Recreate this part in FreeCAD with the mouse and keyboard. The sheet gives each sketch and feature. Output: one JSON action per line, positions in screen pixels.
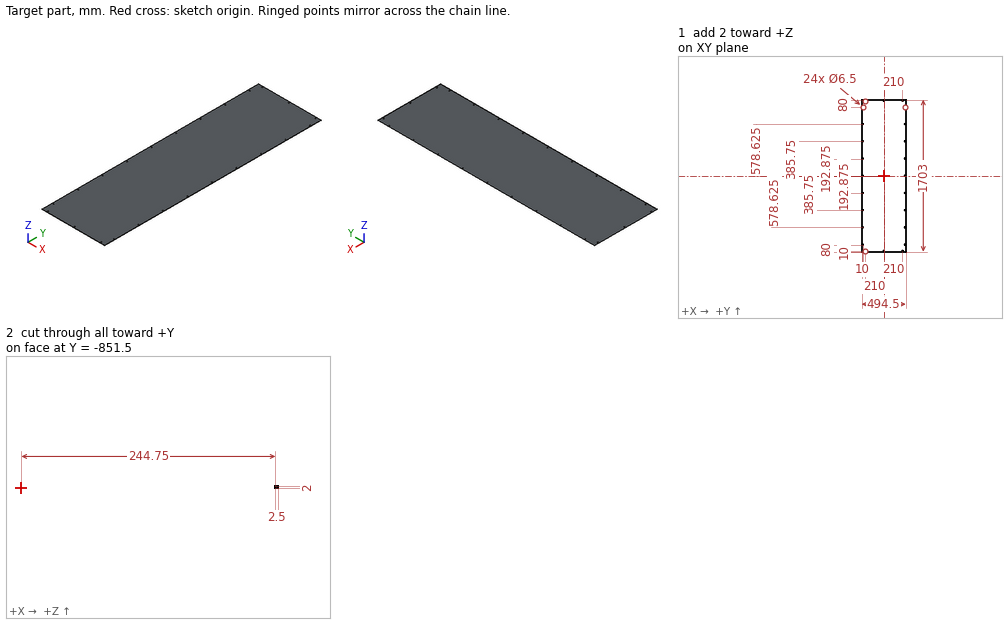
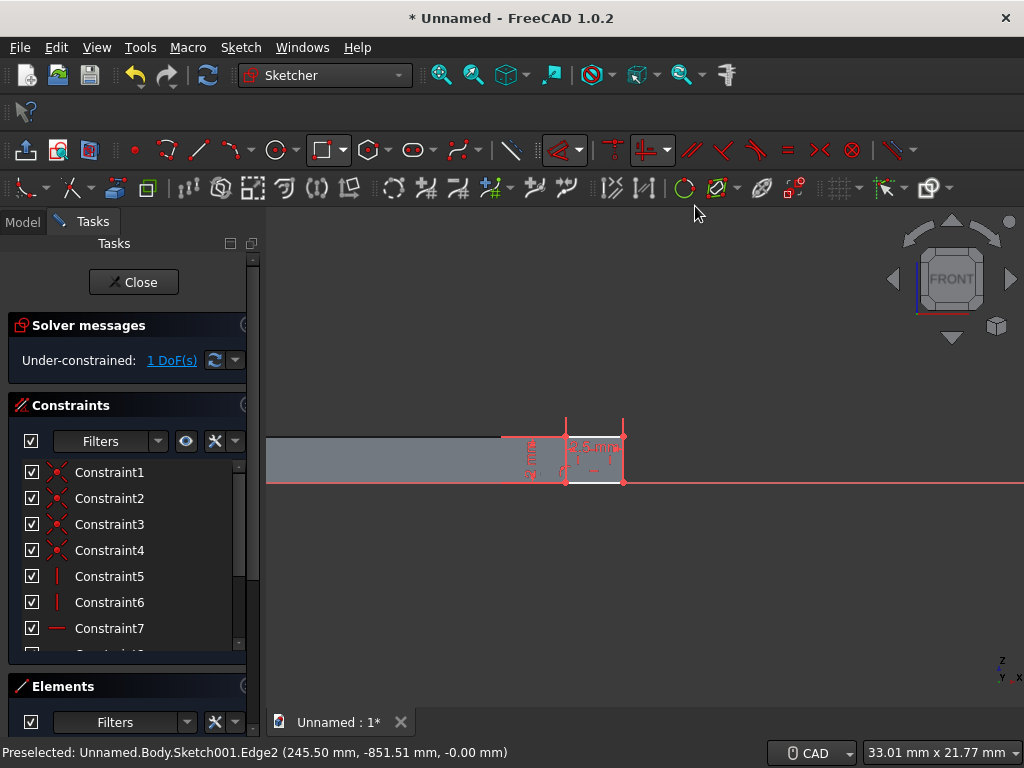
{"action": "scroll", "coordinate": [597, 460], "scroll_direction": "up", "scroll_amount": 10}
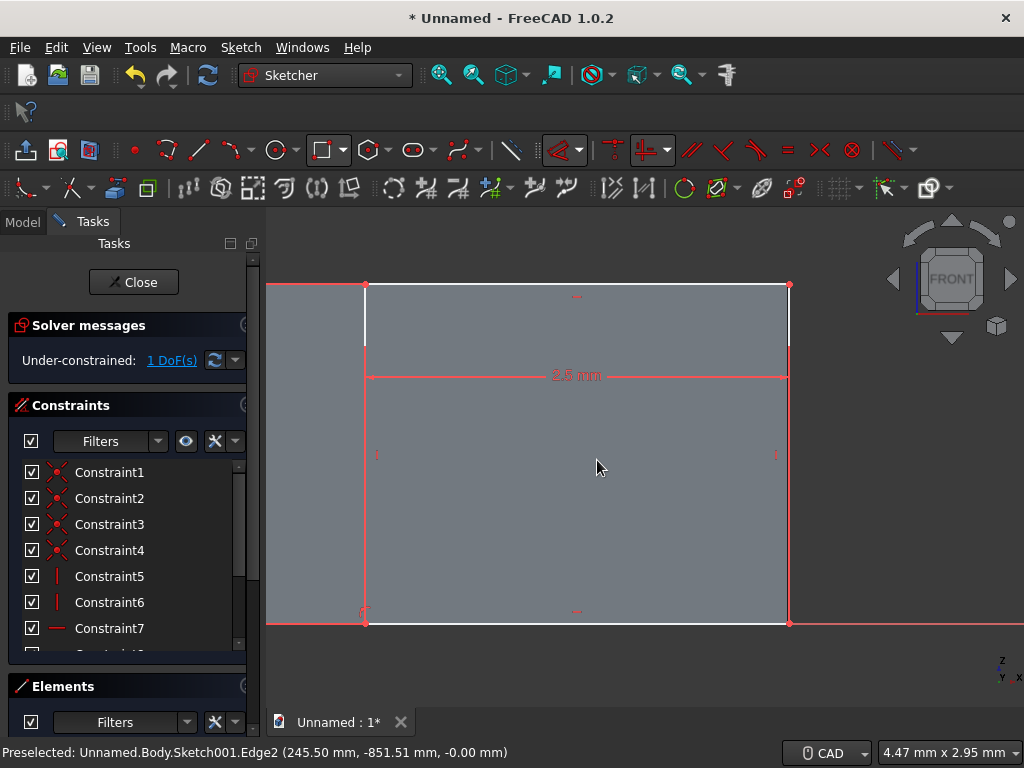
{"action": "left_click", "coordinate": [365, 284]}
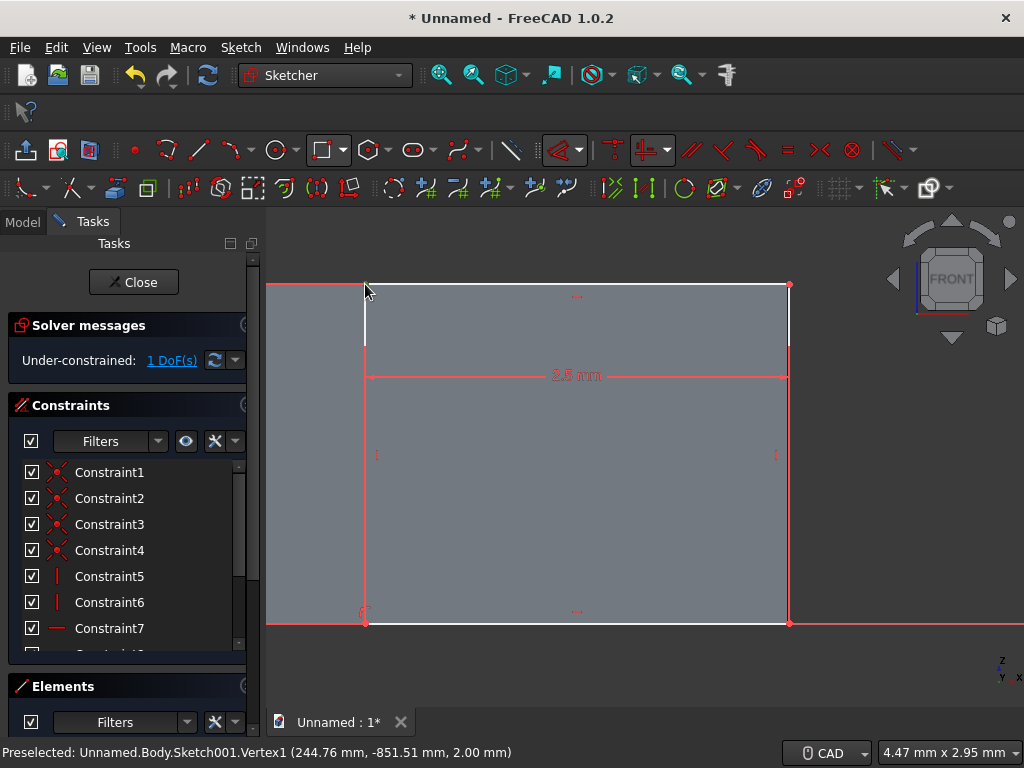
{"action": "key", "text": "l"}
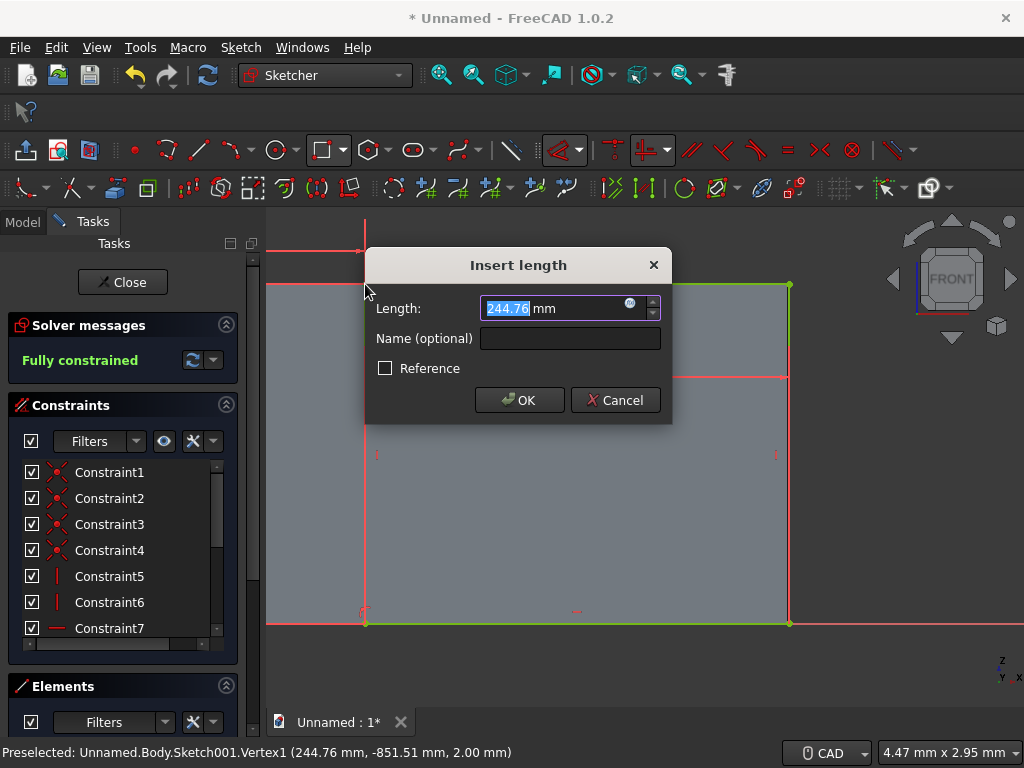
{"action": "type", "text": "244.75"}
{"action": "key", "text": "Return"}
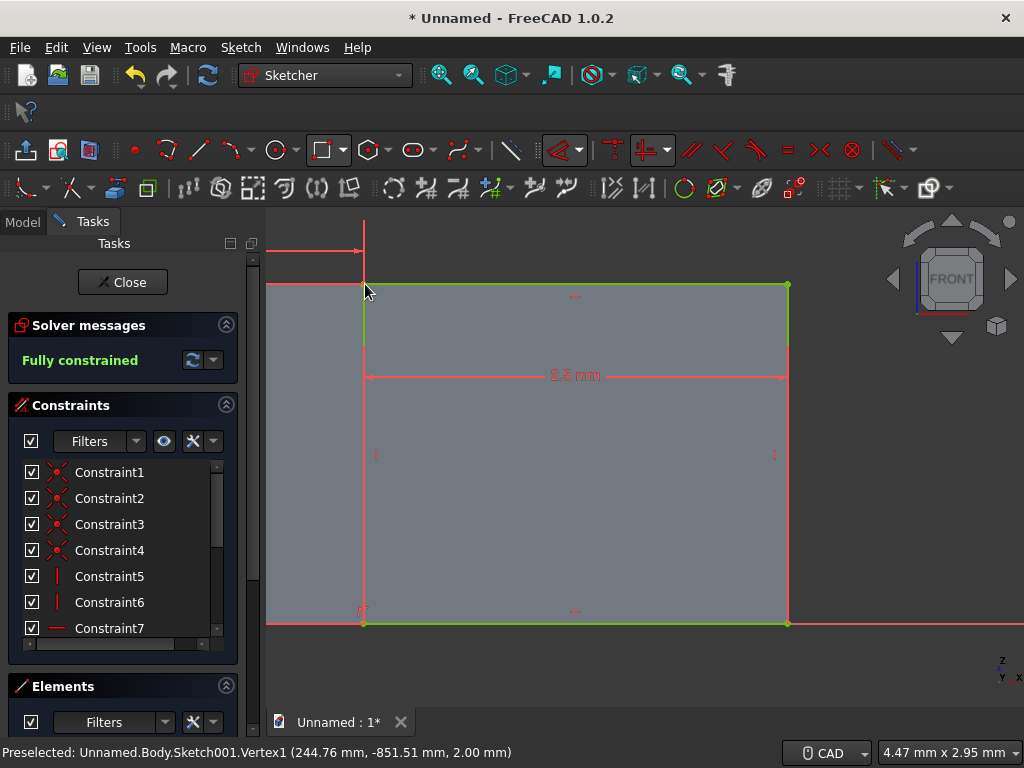
{"action": "left_click", "coordinate": [123, 282]}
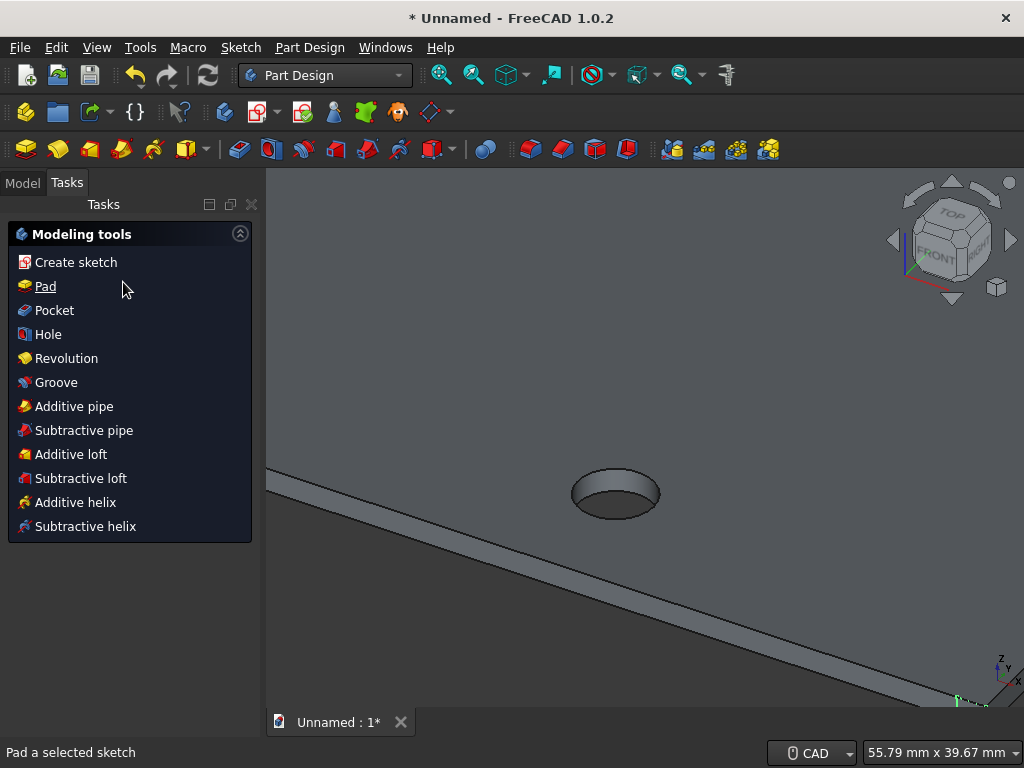
{"action": "left_click", "coordinate": [240, 150]}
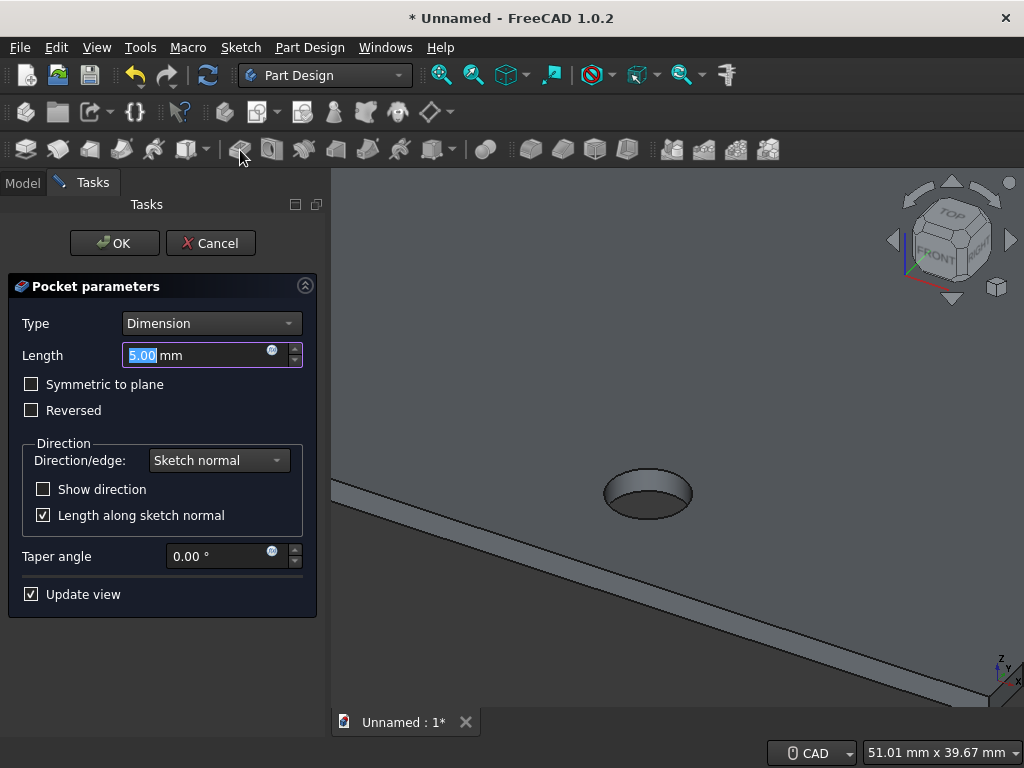
{"action": "left_click", "coordinate": [212, 324]}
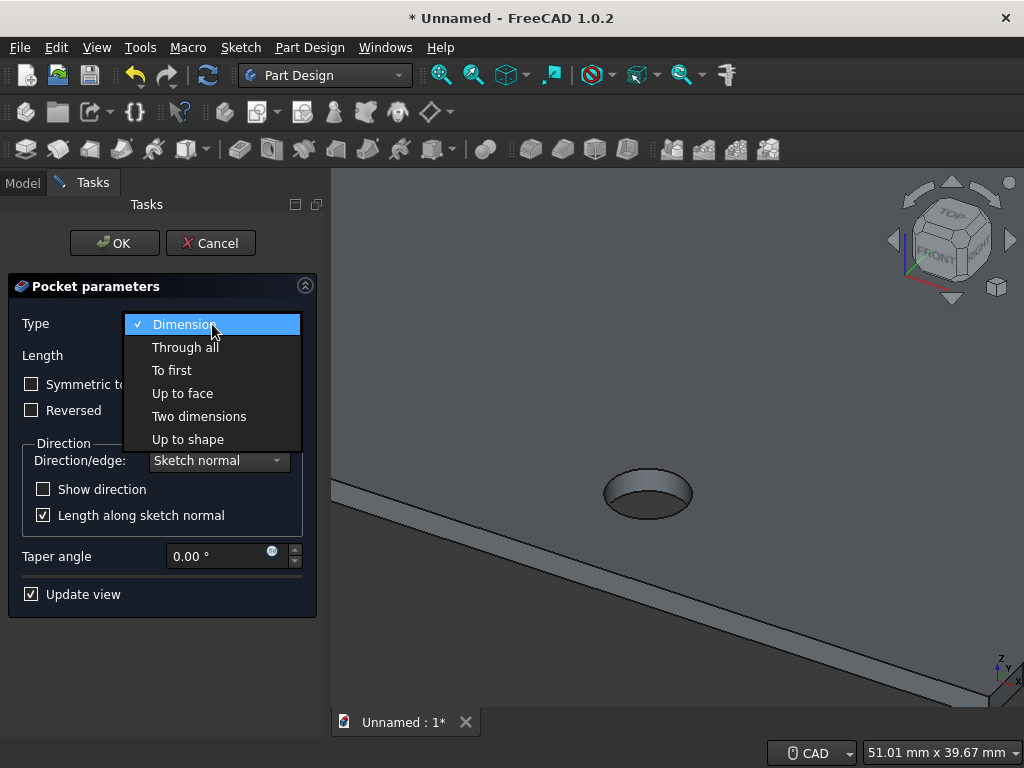
{"action": "left_click", "coordinate": [212, 348]}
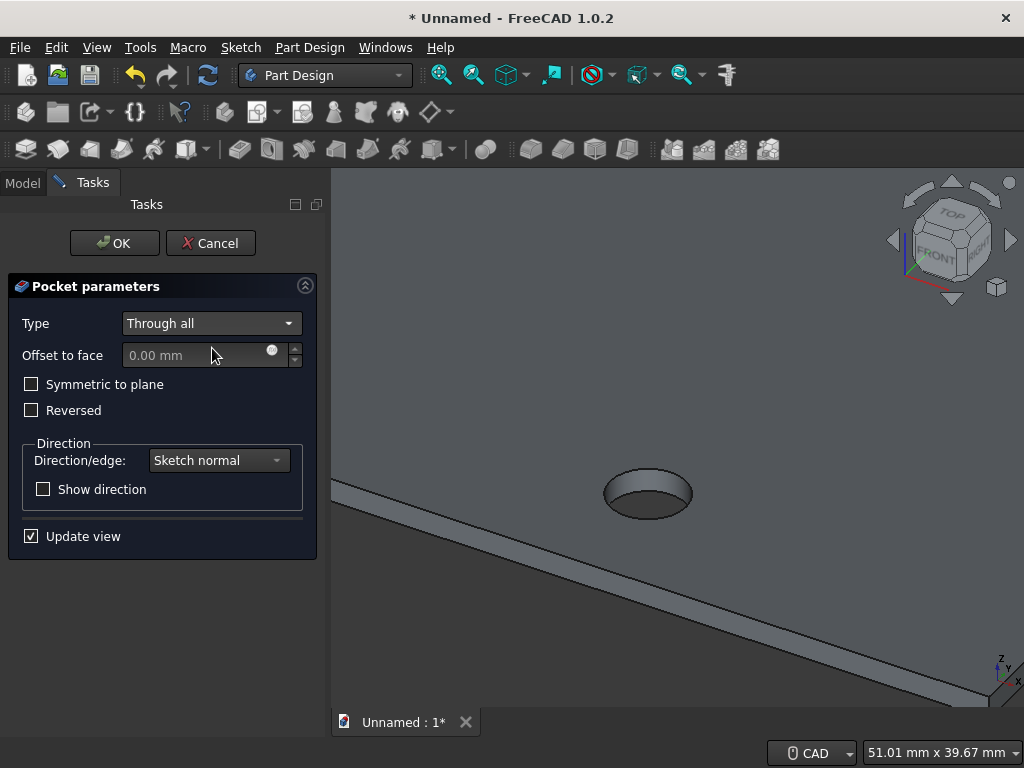
{"action": "left_click", "coordinate": [115, 243]}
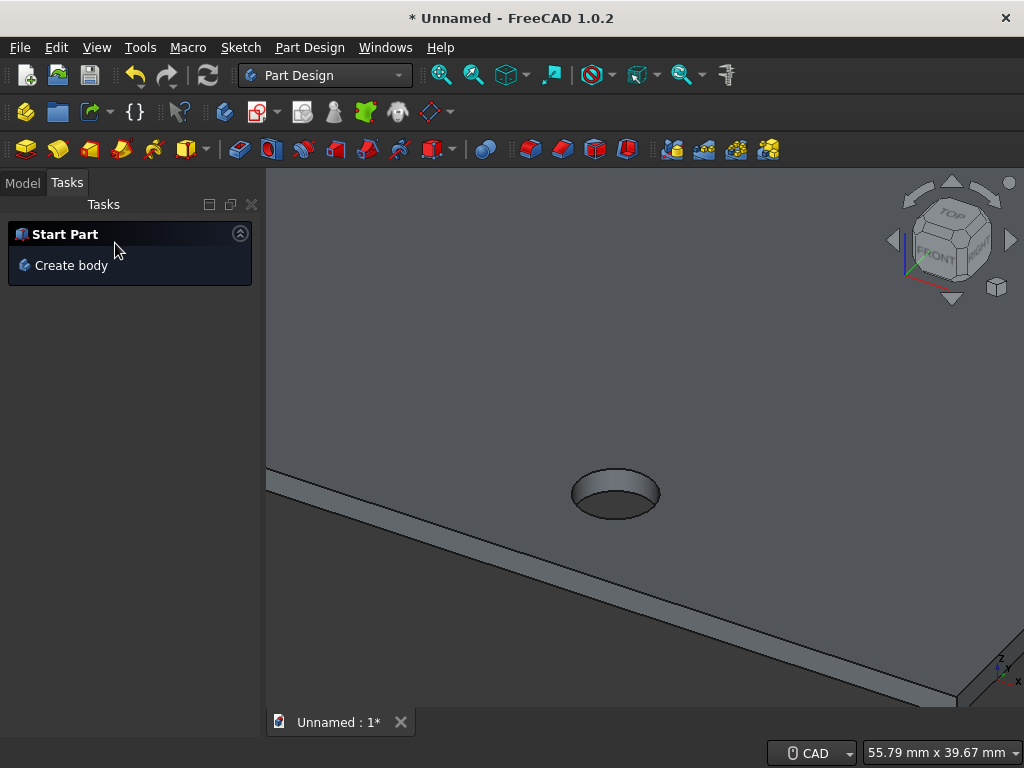
{"action": "key", "text": "0"}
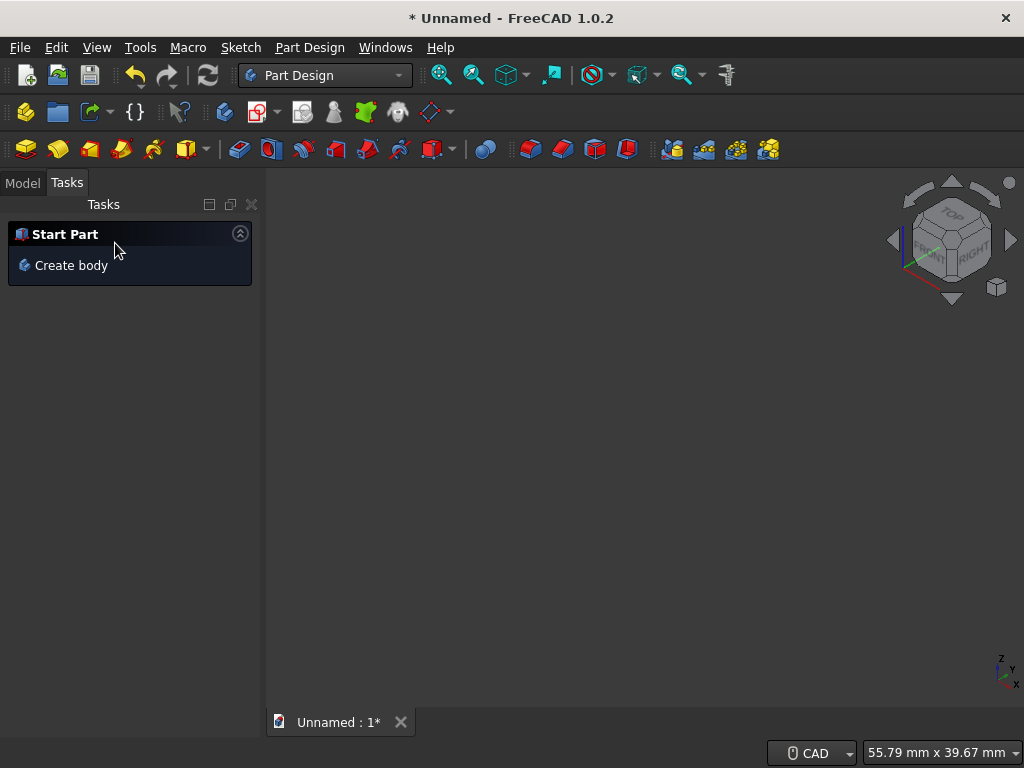
{"action": "left_click", "coordinate": [442, 76]}